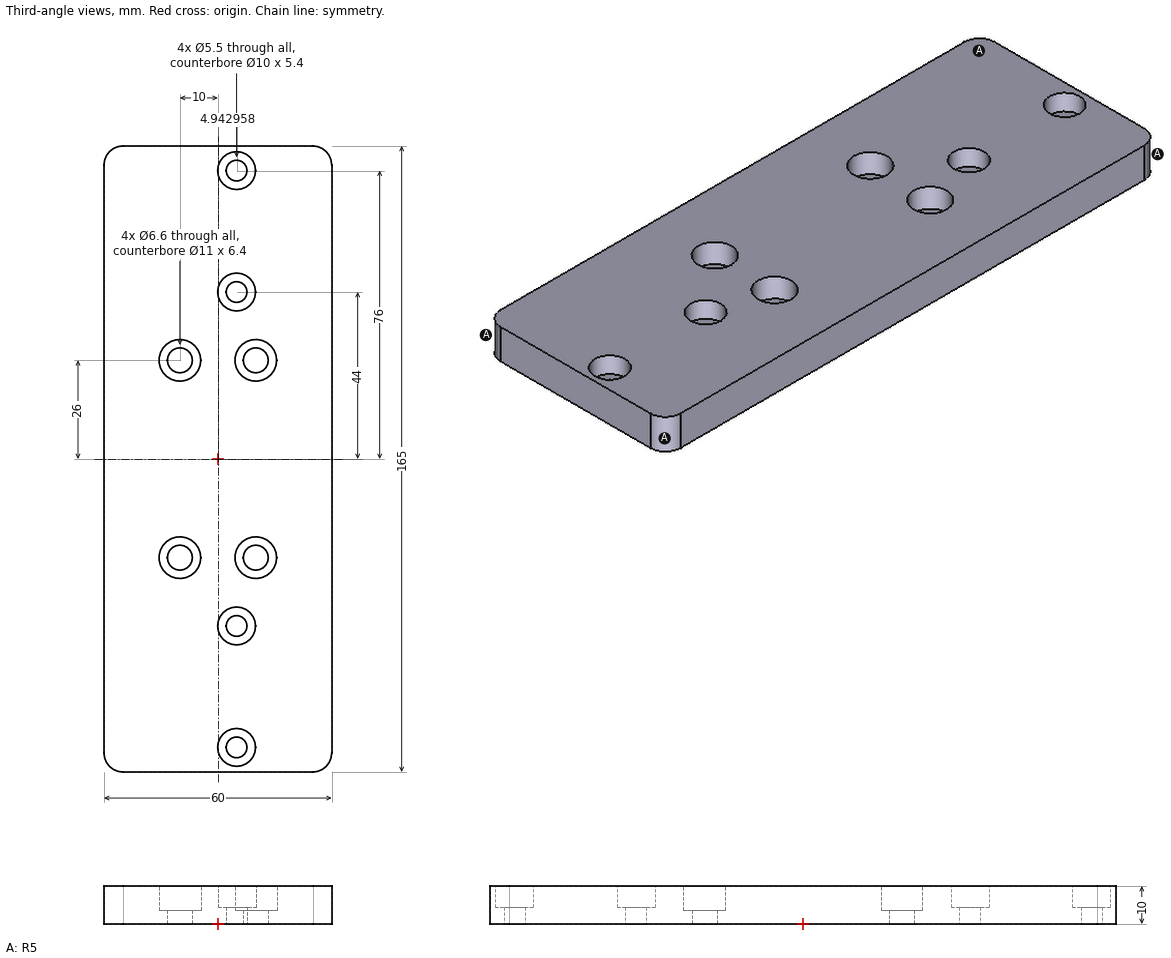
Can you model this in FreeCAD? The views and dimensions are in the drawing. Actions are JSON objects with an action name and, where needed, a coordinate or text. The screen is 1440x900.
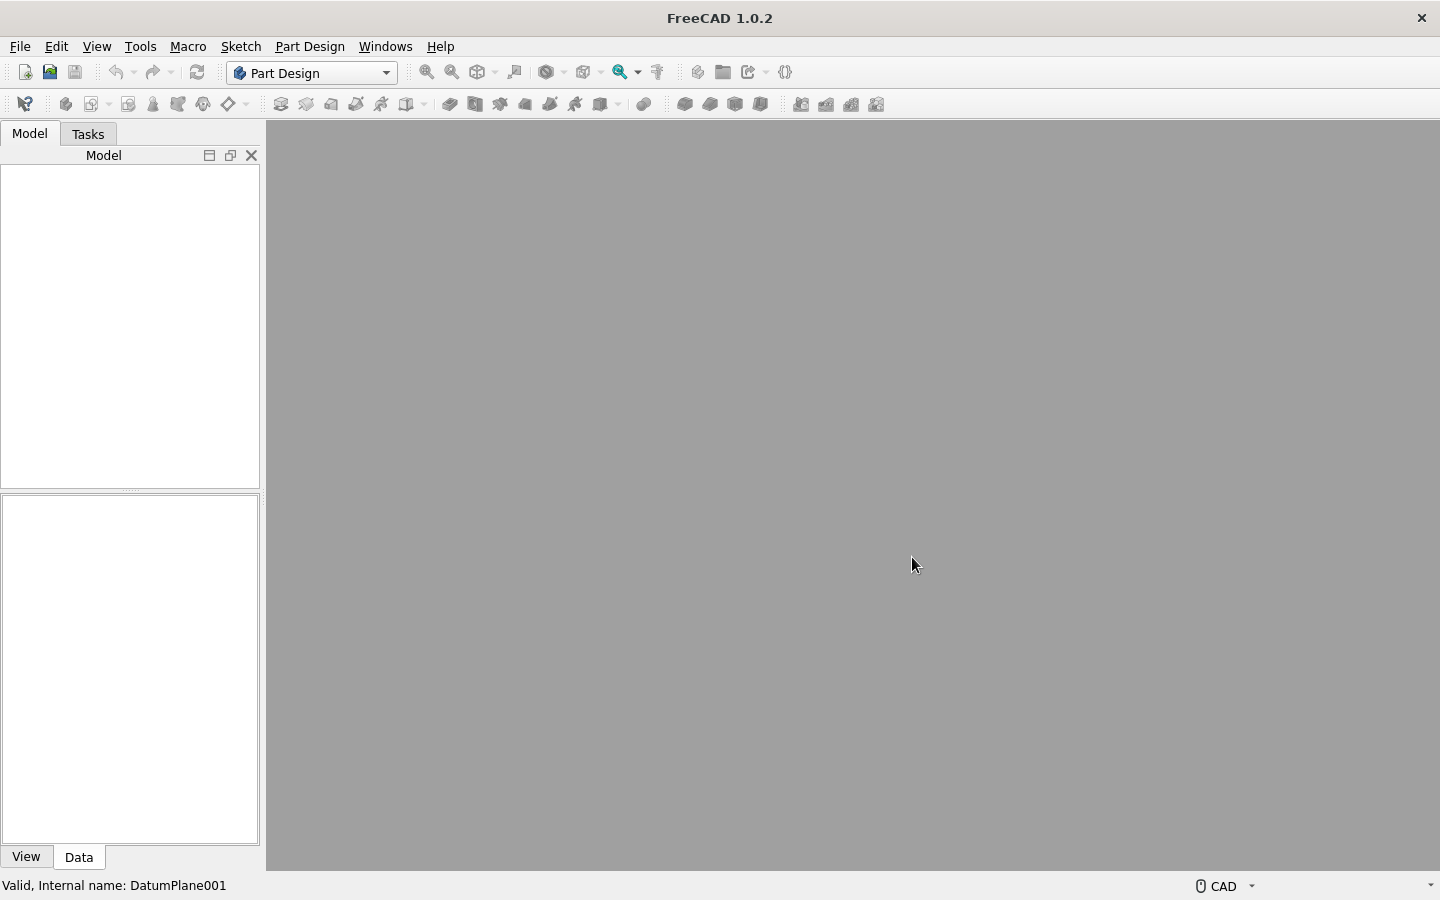
{"action": "left_click", "coordinate": [25, 72]}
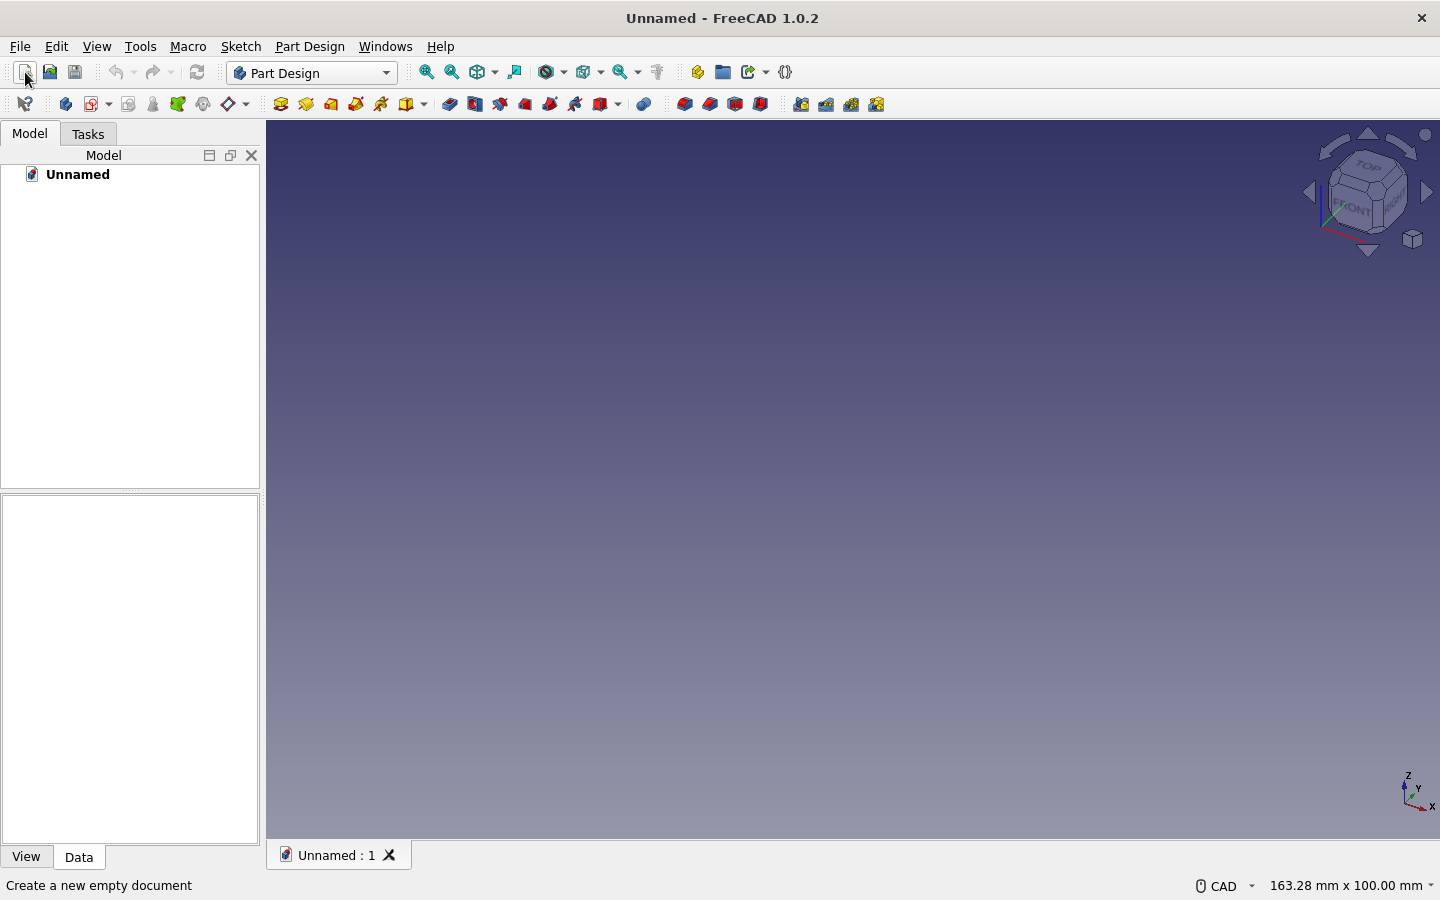
{"action": "left_click", "coordinate": [90, 104]}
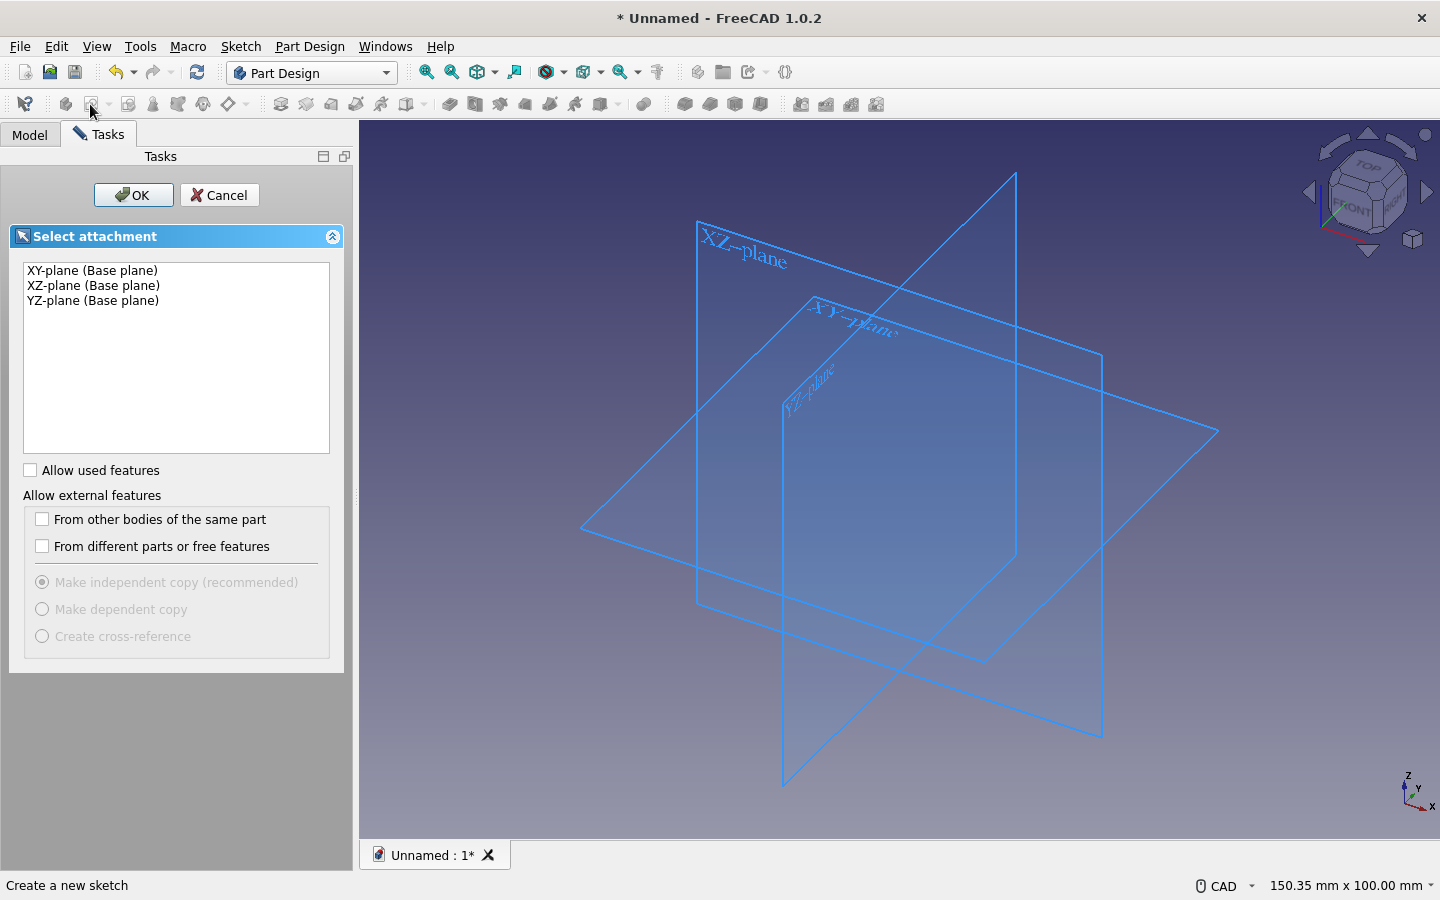
{"action": "left_click", "coordinate": [84, 270]}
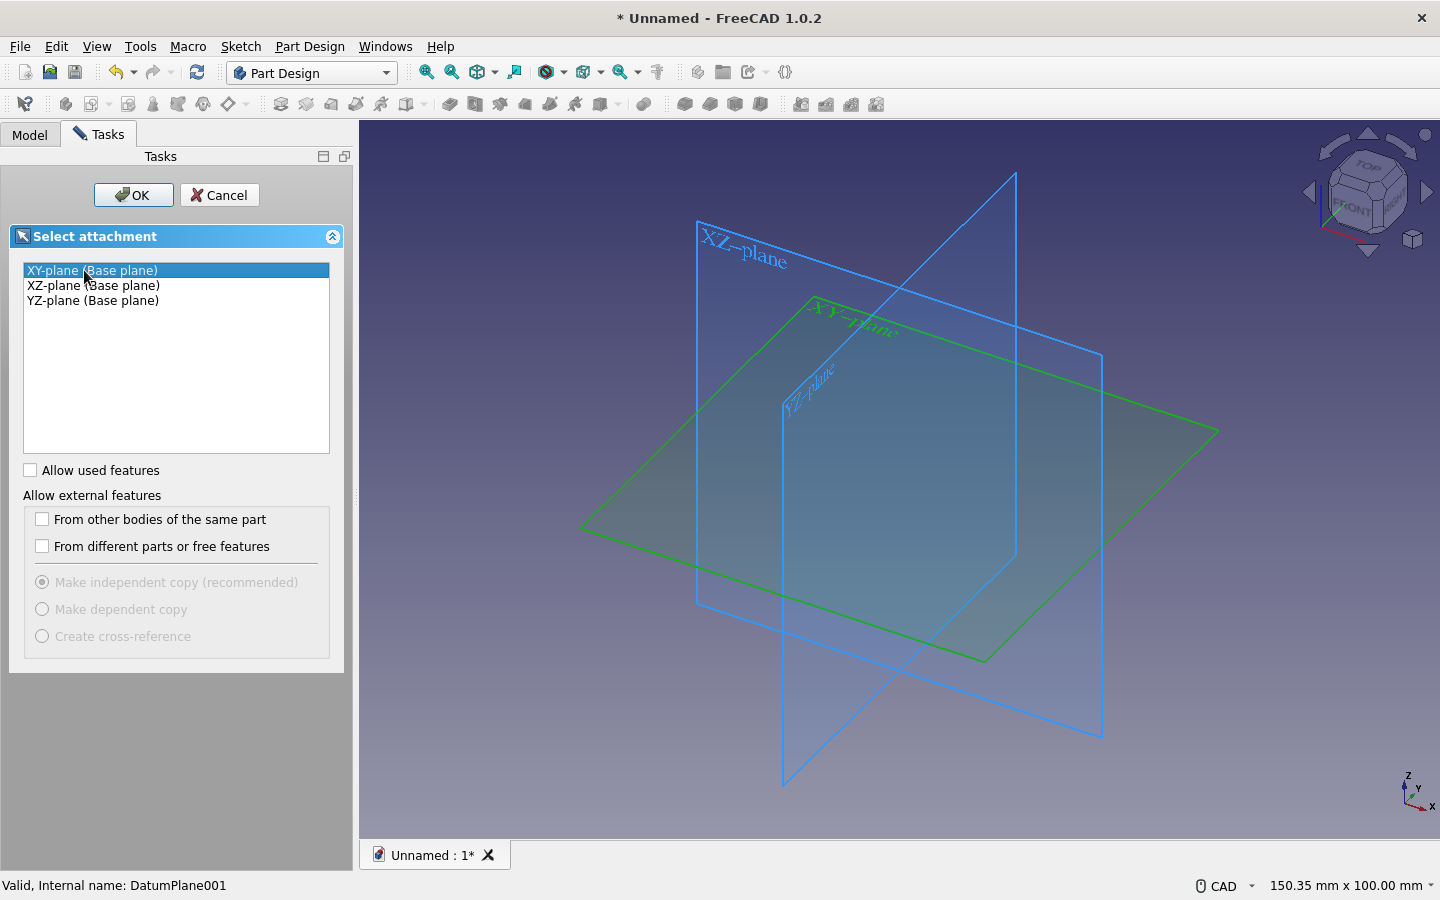
{"action": "left_click", "coordinate": [134, 195]}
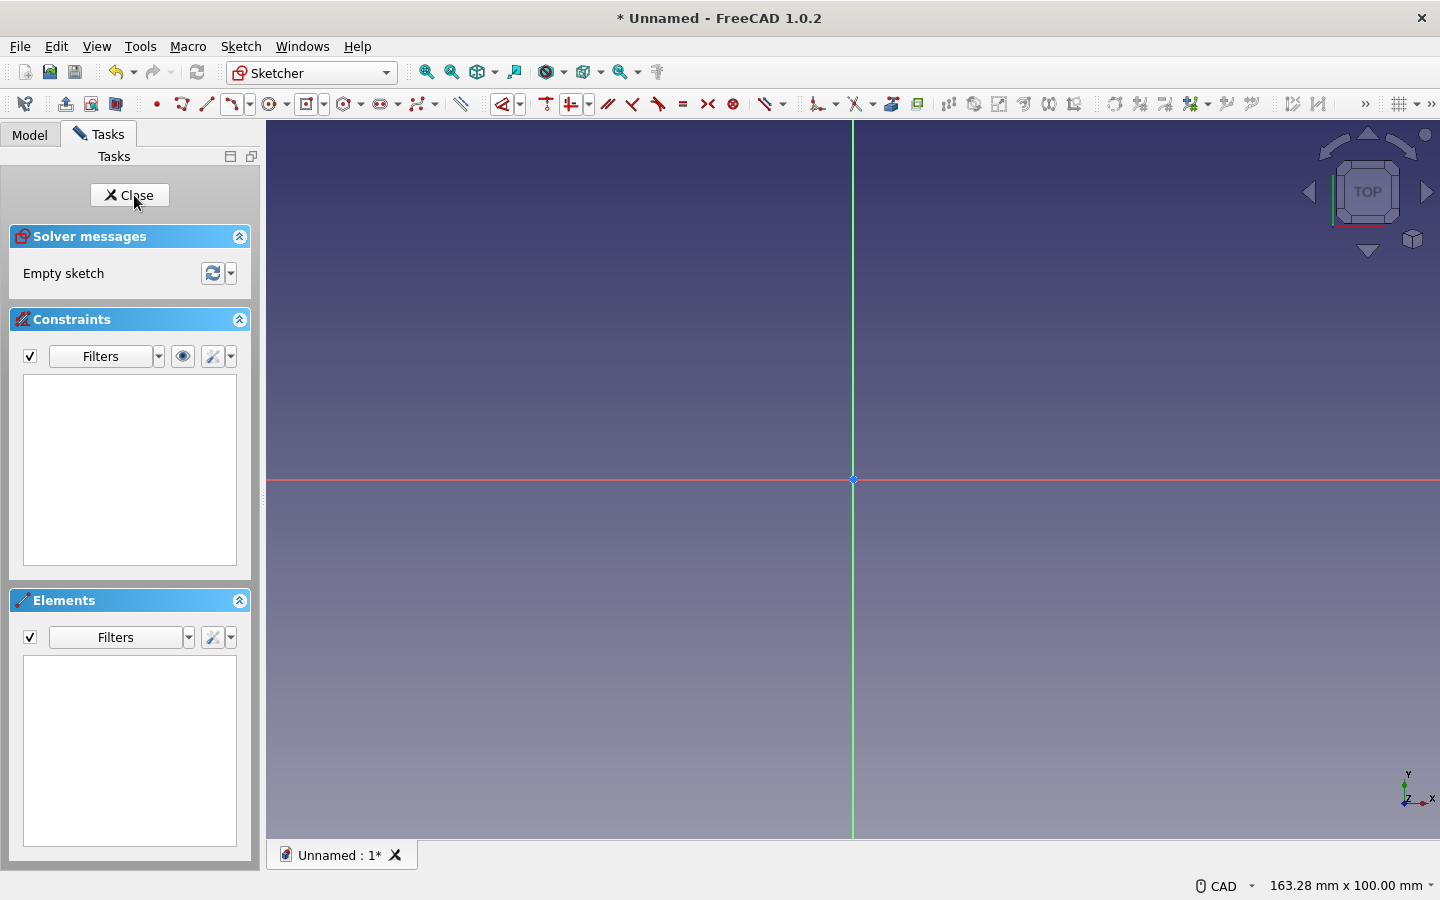
{"action": "scroll", "coordinate": [745, 480], "scroll_direction": "down", "scroll_amount": 5}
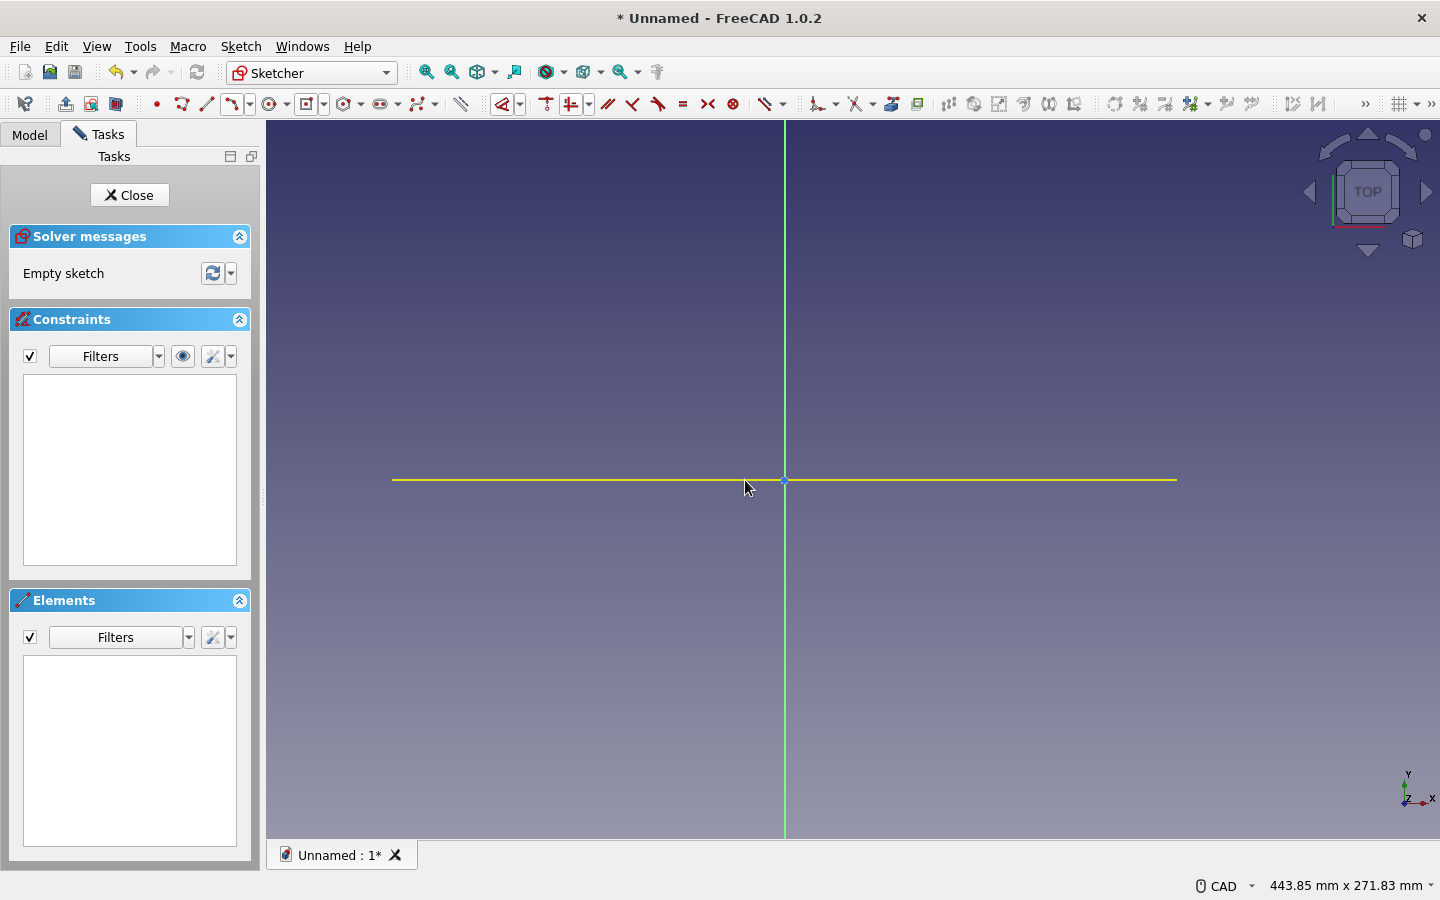
{"action": "left_click", "coordinate": [306, 104]}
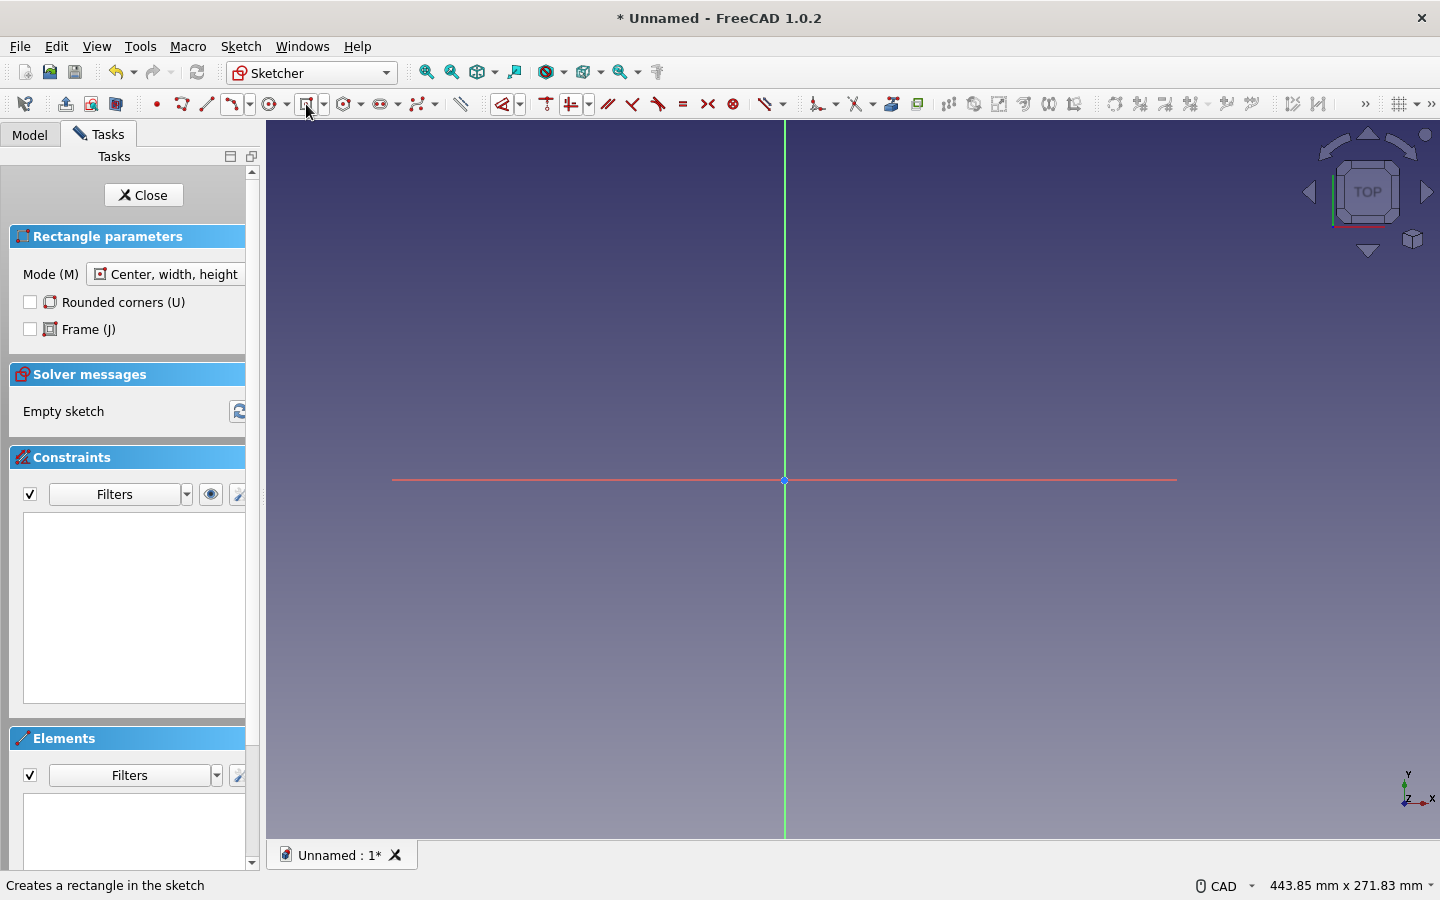
{"action": "left_click", "coordinate": [785, 480]}
{"action": "left_click", "coordinate": [864, 262]}
{"action": "key", "text": "Escape"}